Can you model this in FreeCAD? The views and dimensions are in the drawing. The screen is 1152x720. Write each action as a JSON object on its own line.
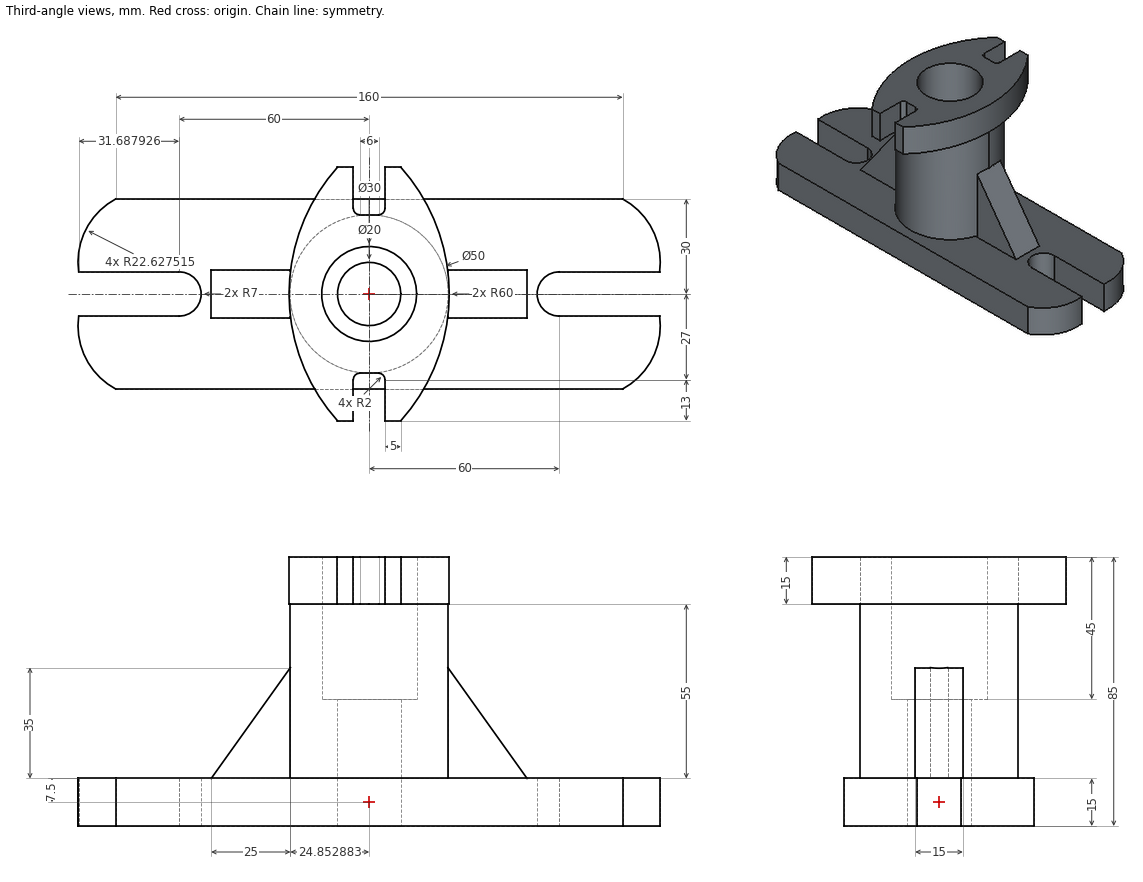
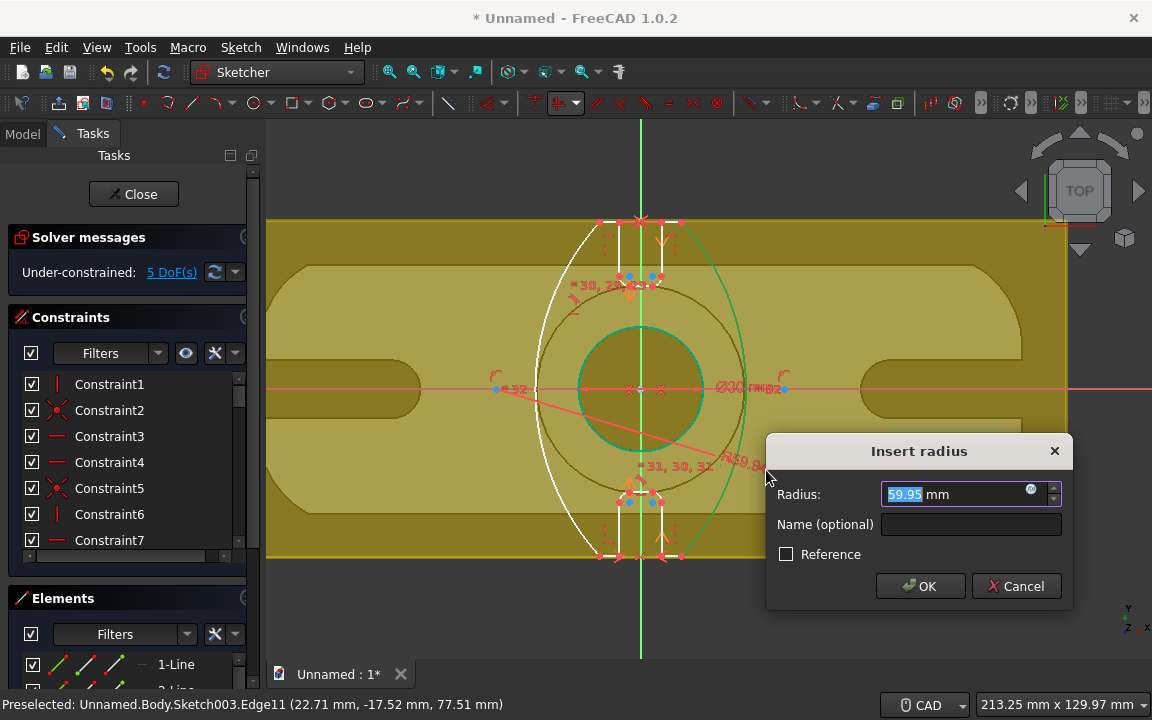
{"action": "type", "text": "60"}
{"action": "key", "text": "Return"}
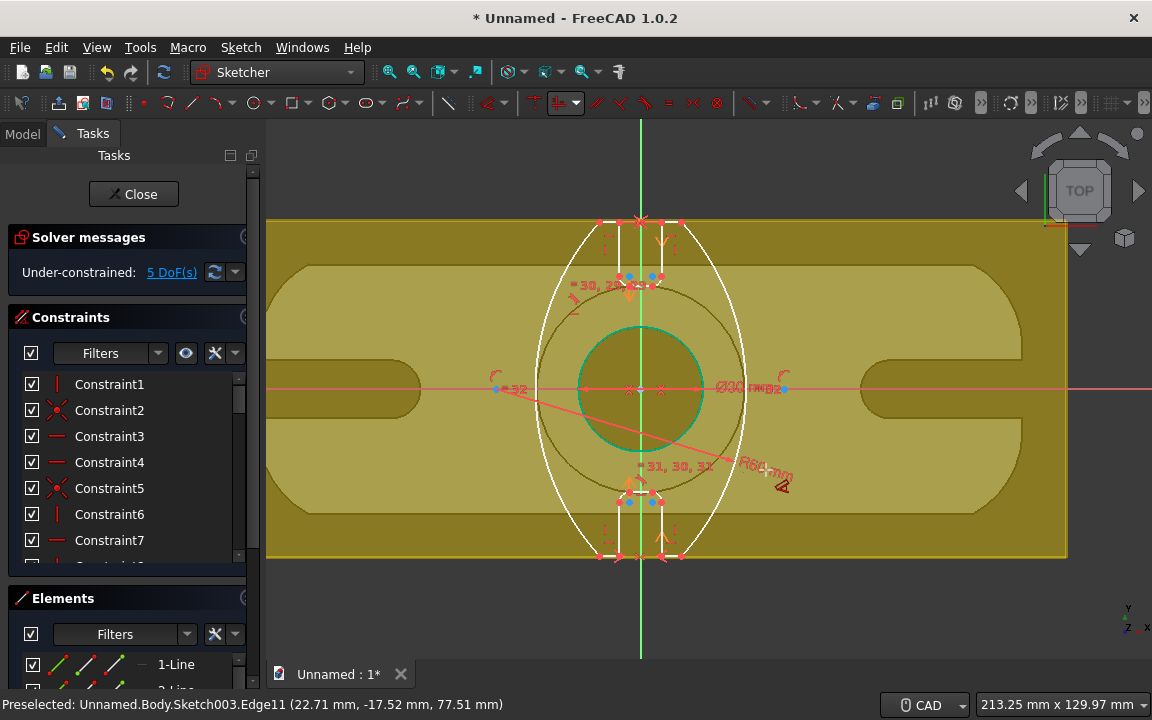
{"action": "scroll", "coordinate": [659, 283], "scroll_direction": "up", "scroll_amount": 8}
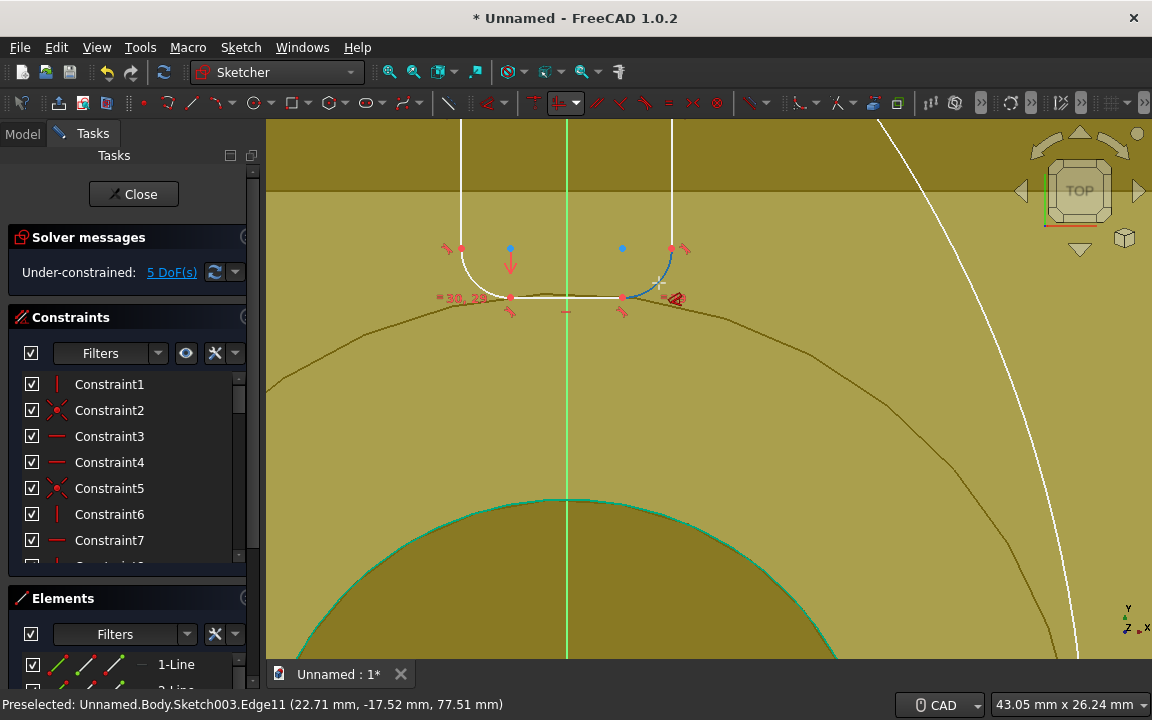
{"action": "left_click", "coordinate": [657, 283]}
{"action": "left_click", "coordinate": [680, 306]}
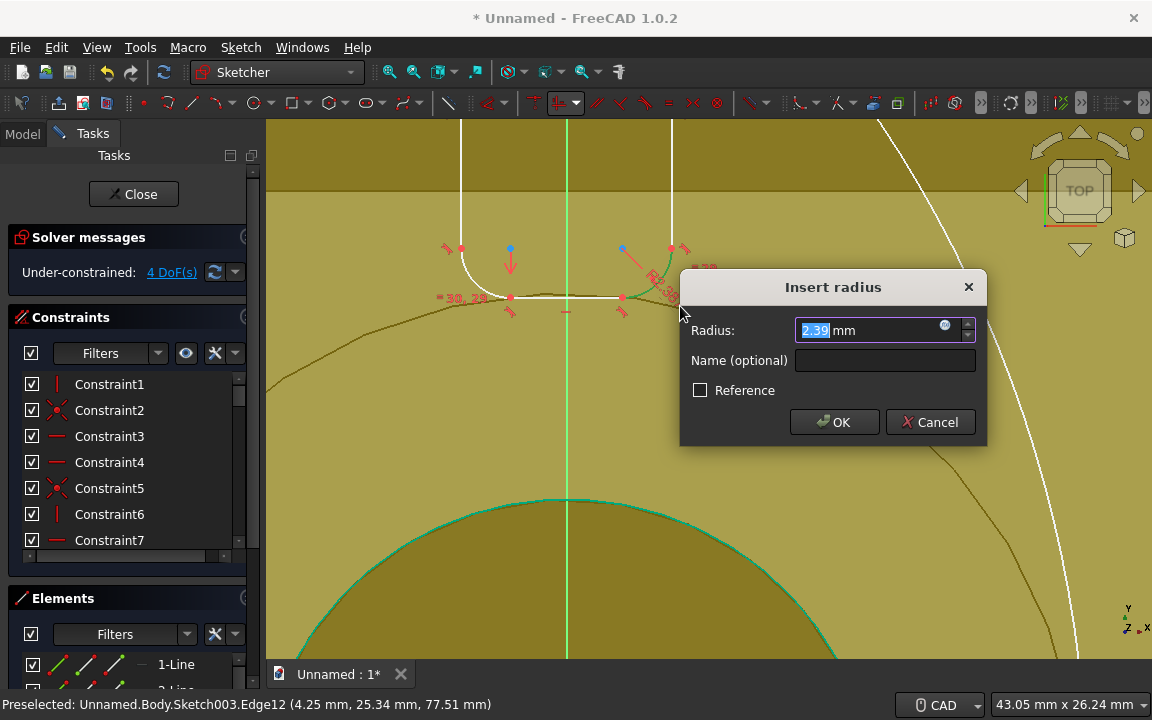
{"action": "type", "text": "2"}
{"action": "key", "text": "Return"}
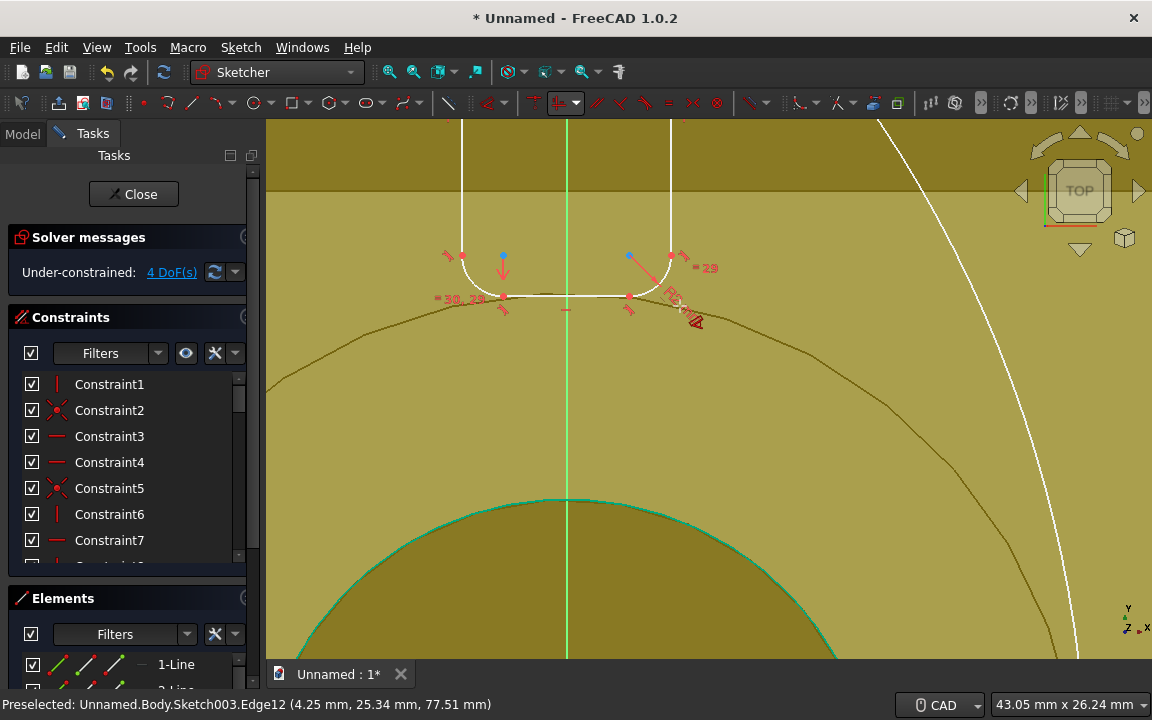
{"action": "scroll", "coordinate": [659, 283], "scroll_direction": "down", "scroll_amount": 8}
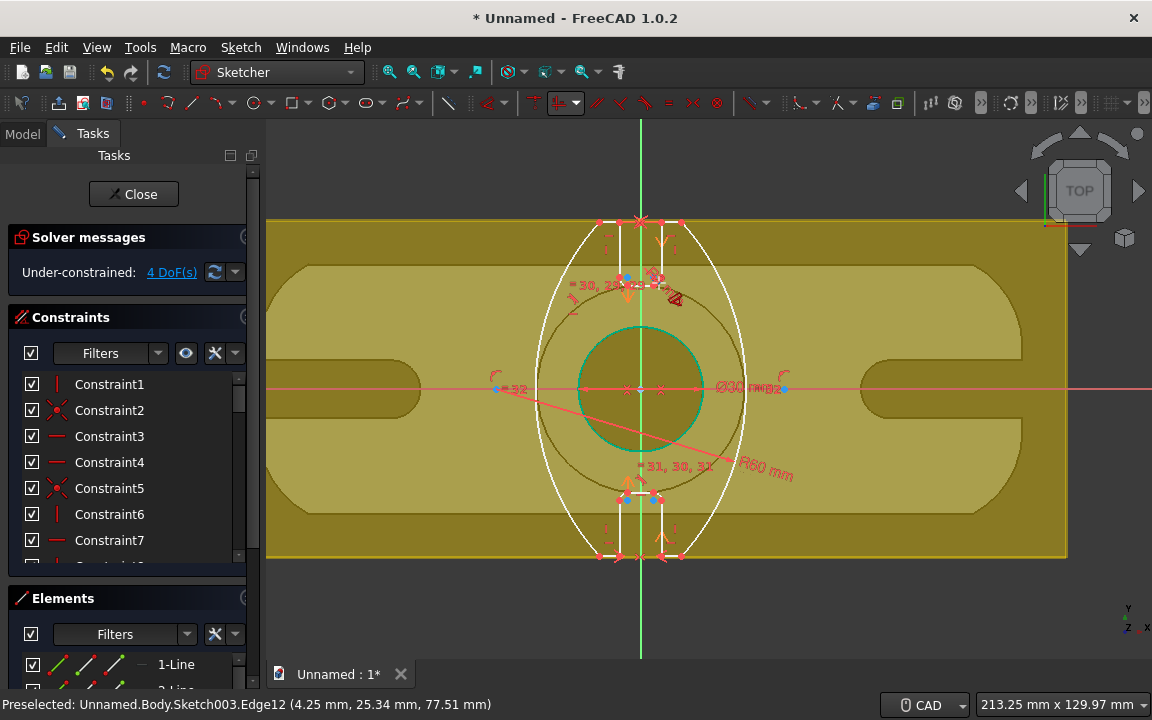
{"action": "scroll", "coordinate": [668, 556], "scroll_direction": "up", "scroll_amount": 5}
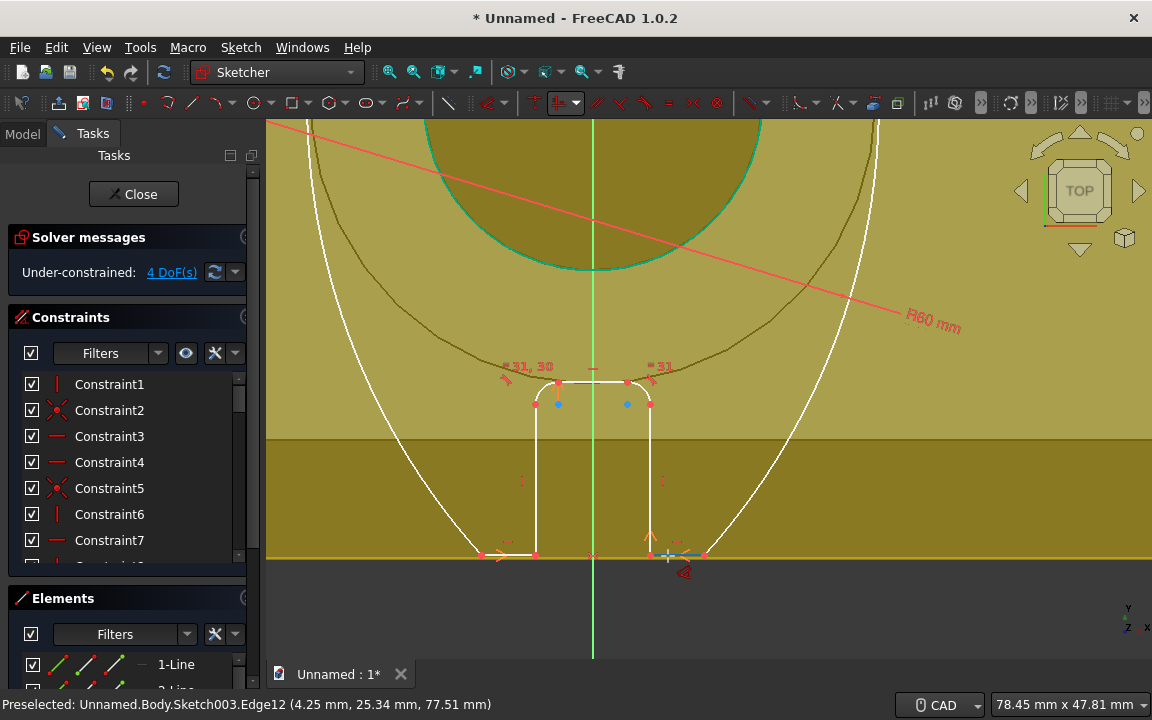
{"action": "left_click", "coordinate": [667, 555]}
{"action": "left_click", "coordinate": [677, 589]}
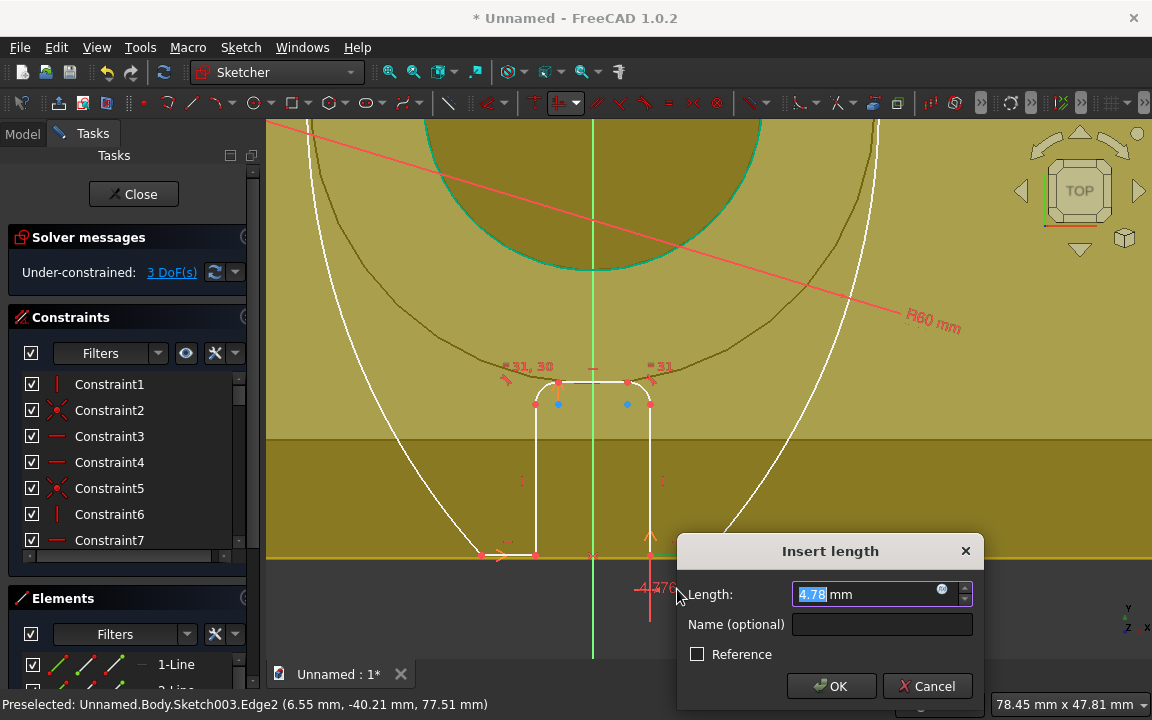
{"action": "type", "text": "5"}
{"action": "key", "text": "Return"}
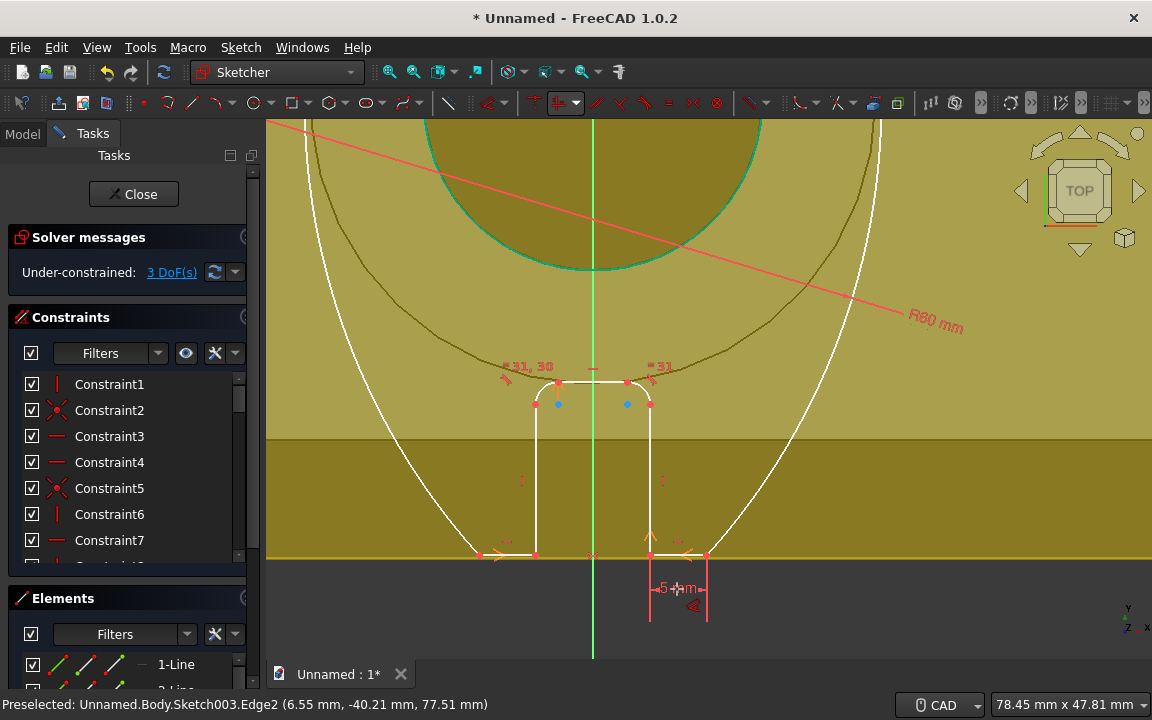
{"action": "scroll", "coordinate": [668, 556], "scroll_direction": "down", "scroll_amount": 5}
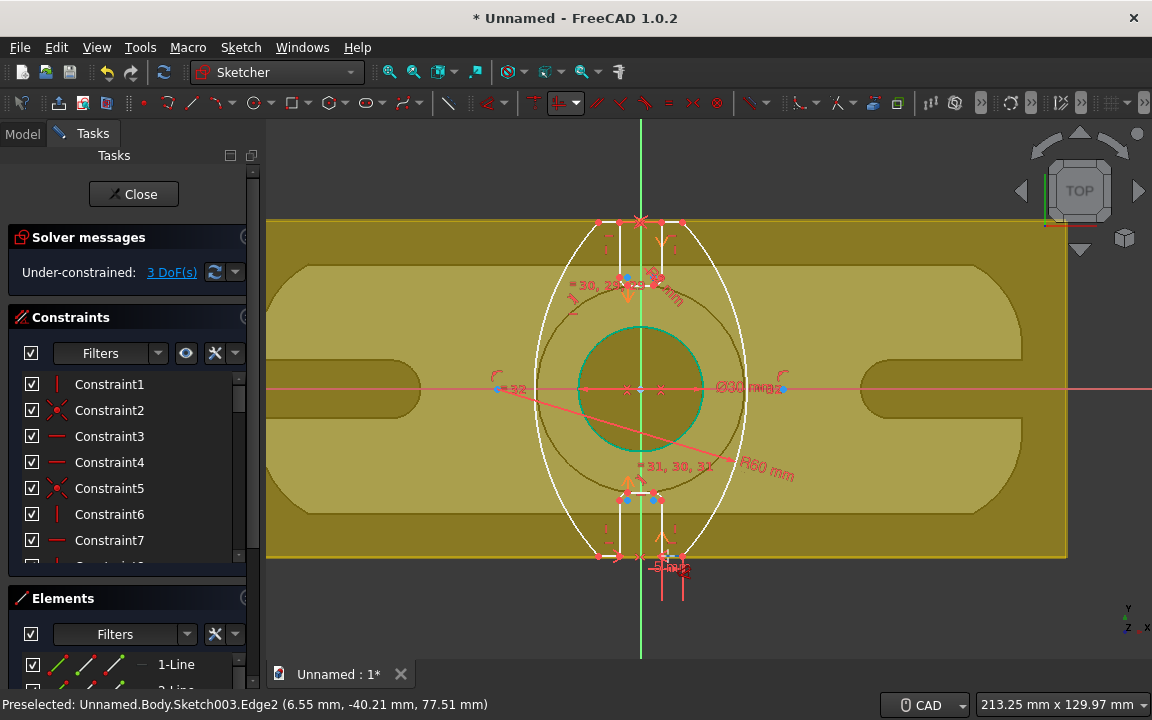
{"action": "scroll", "coordinate": [646, 286], "scroll_direction": "up", "scroll_amount": 5}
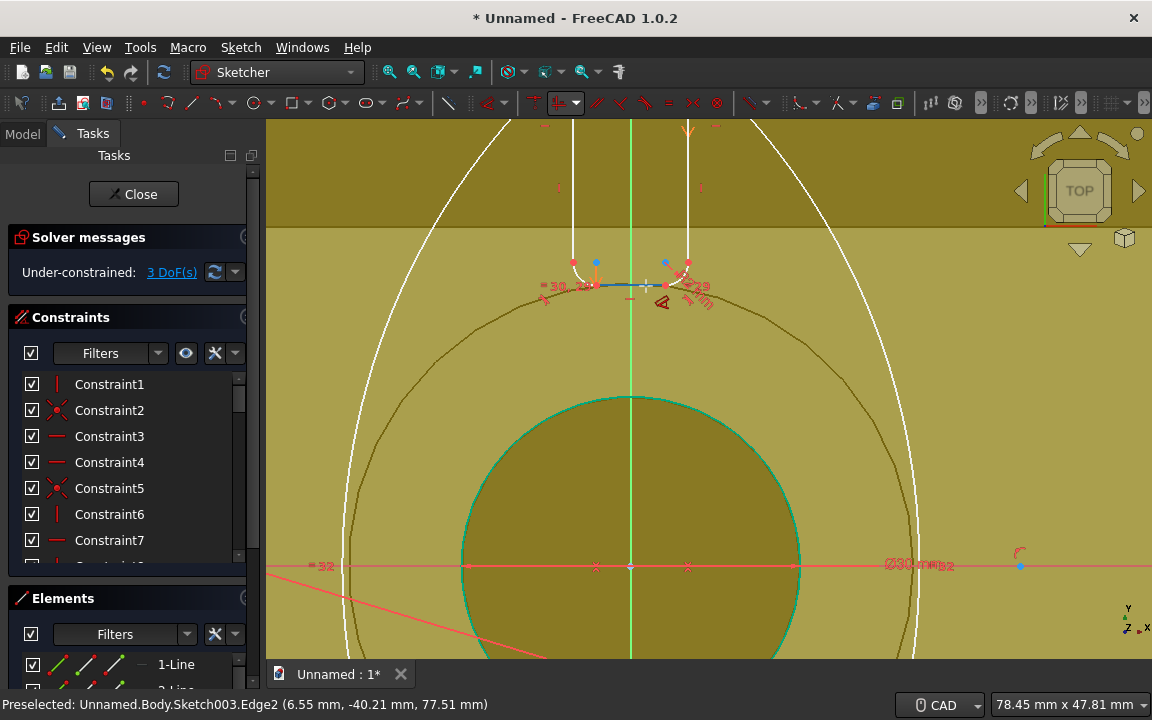
{"action": "left_click", "coordinate": [645, 285]}
{"action": "left_click", "coordinate": [615, 251]}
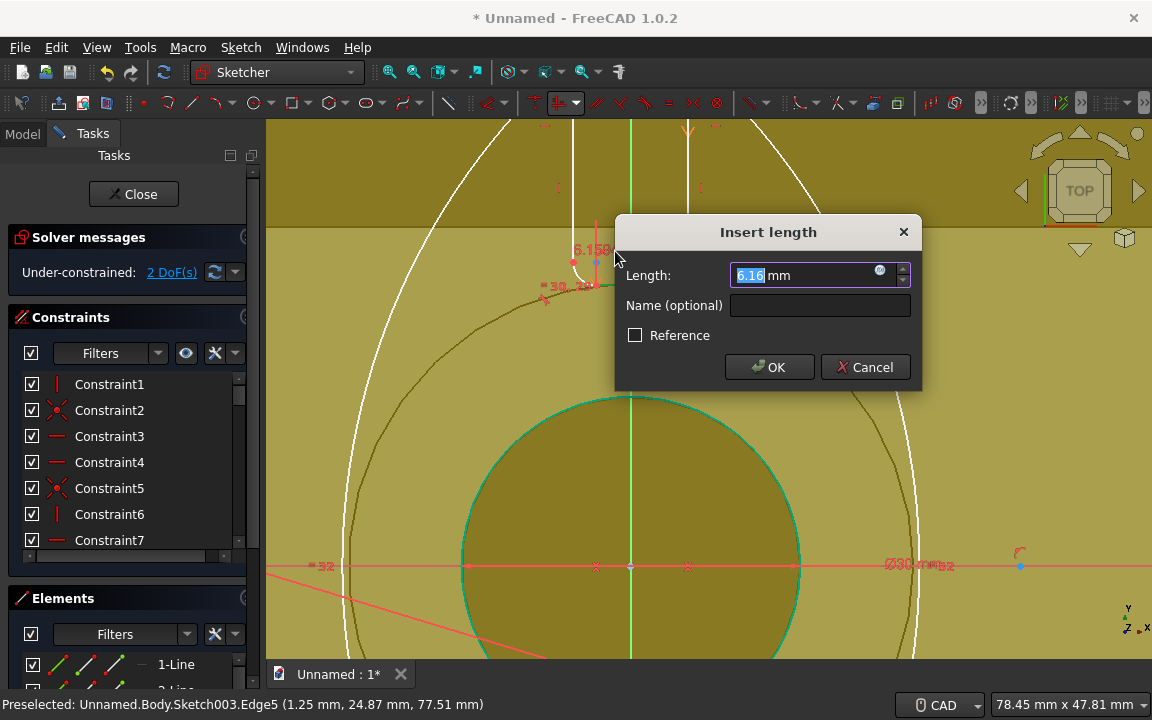
{"action": "type", "text": "6"}
{"action": "key", "text": "Return"}